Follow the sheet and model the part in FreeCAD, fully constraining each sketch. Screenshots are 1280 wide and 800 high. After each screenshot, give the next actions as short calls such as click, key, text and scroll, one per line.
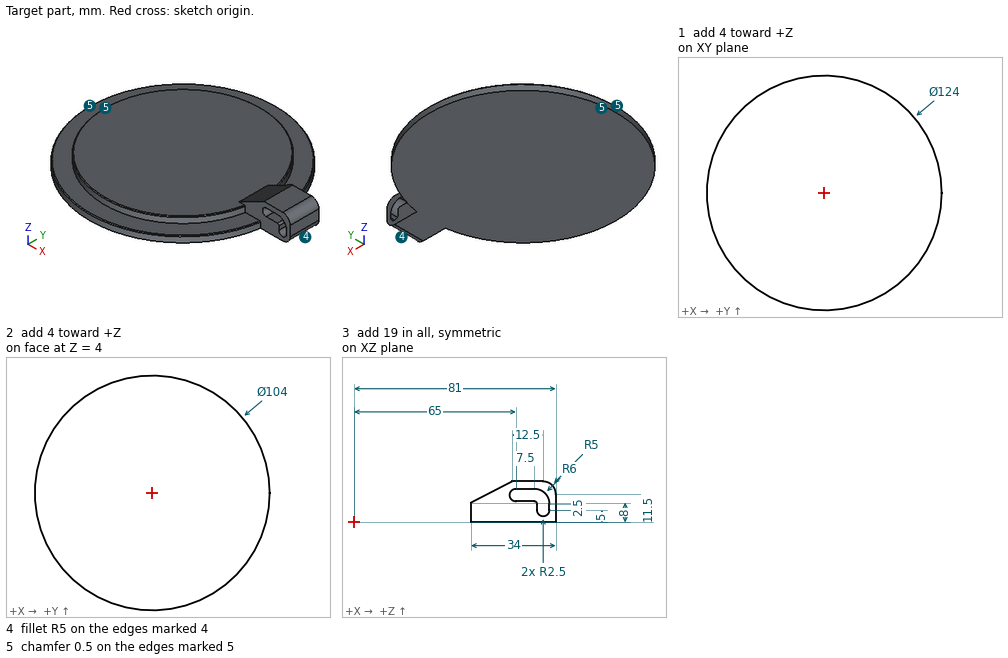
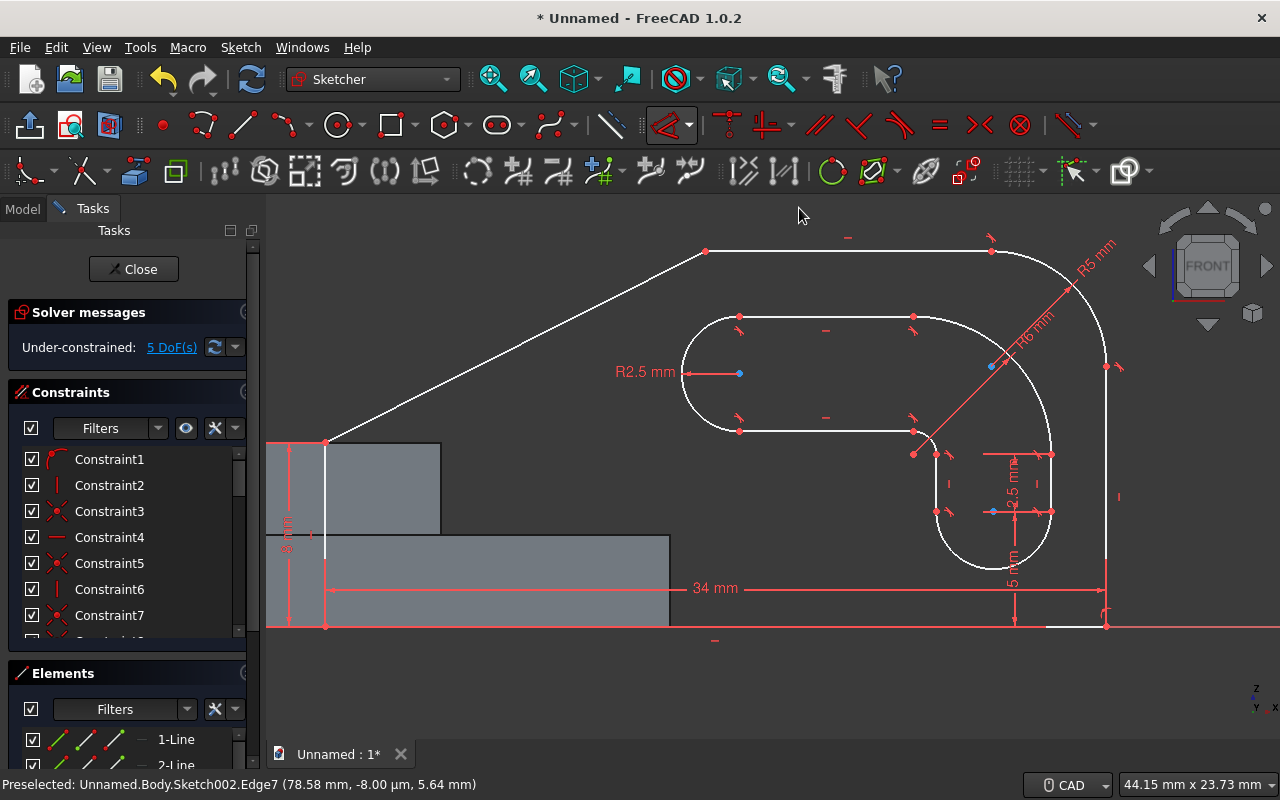
click(861, 317)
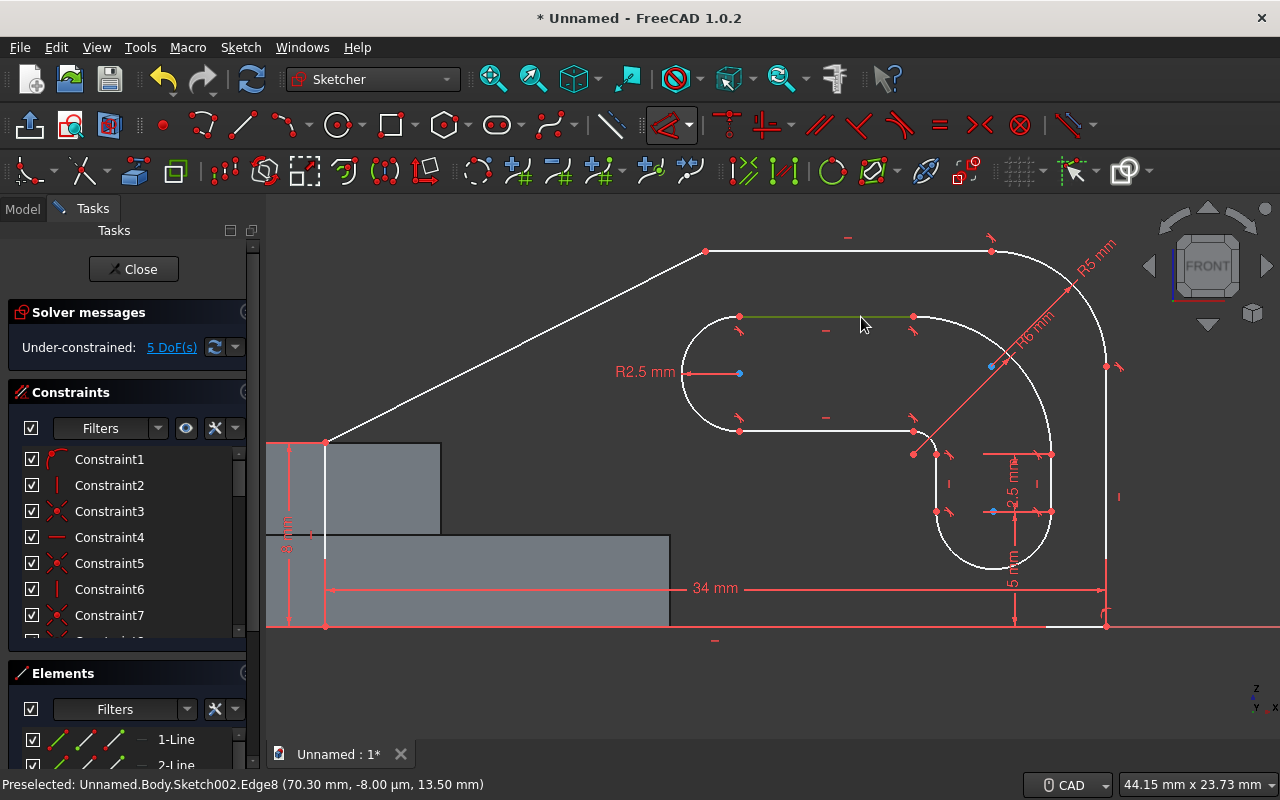
key(l)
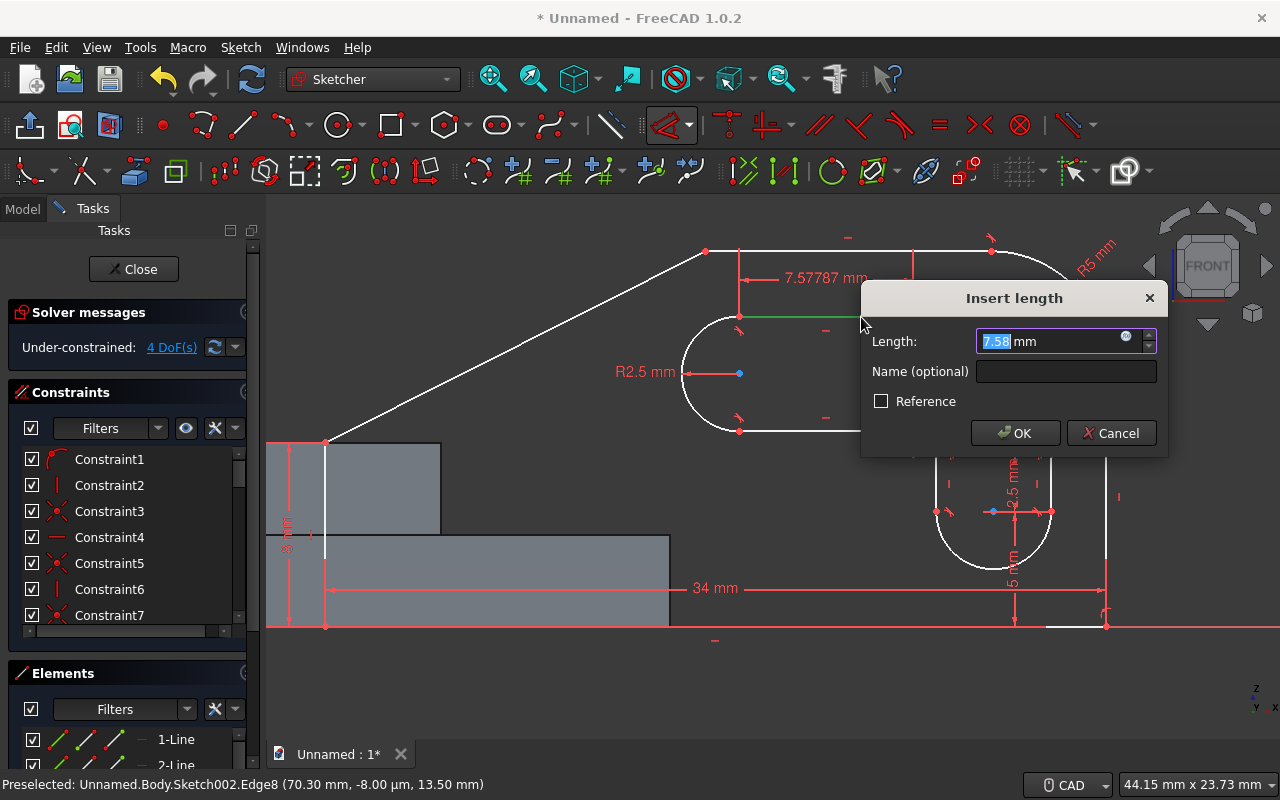
text(7.5)
key(Return)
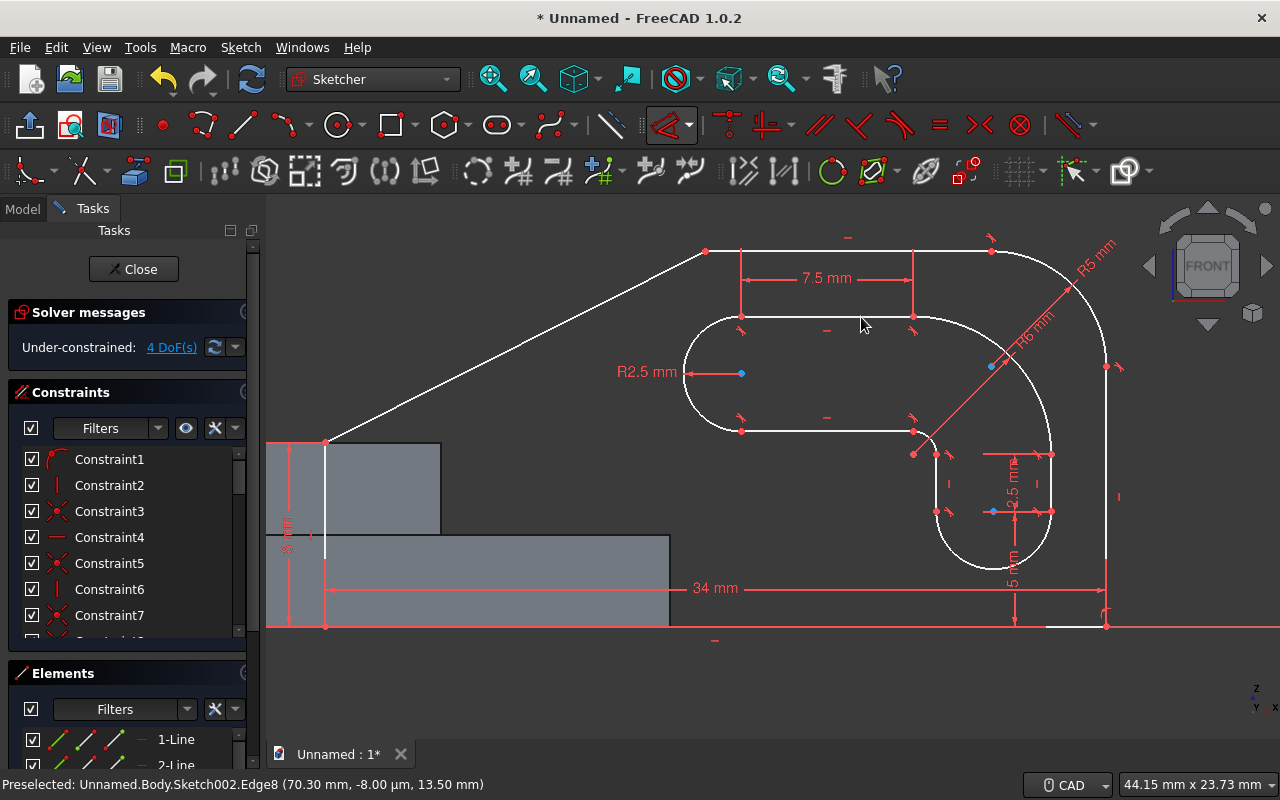
click(1106, 366)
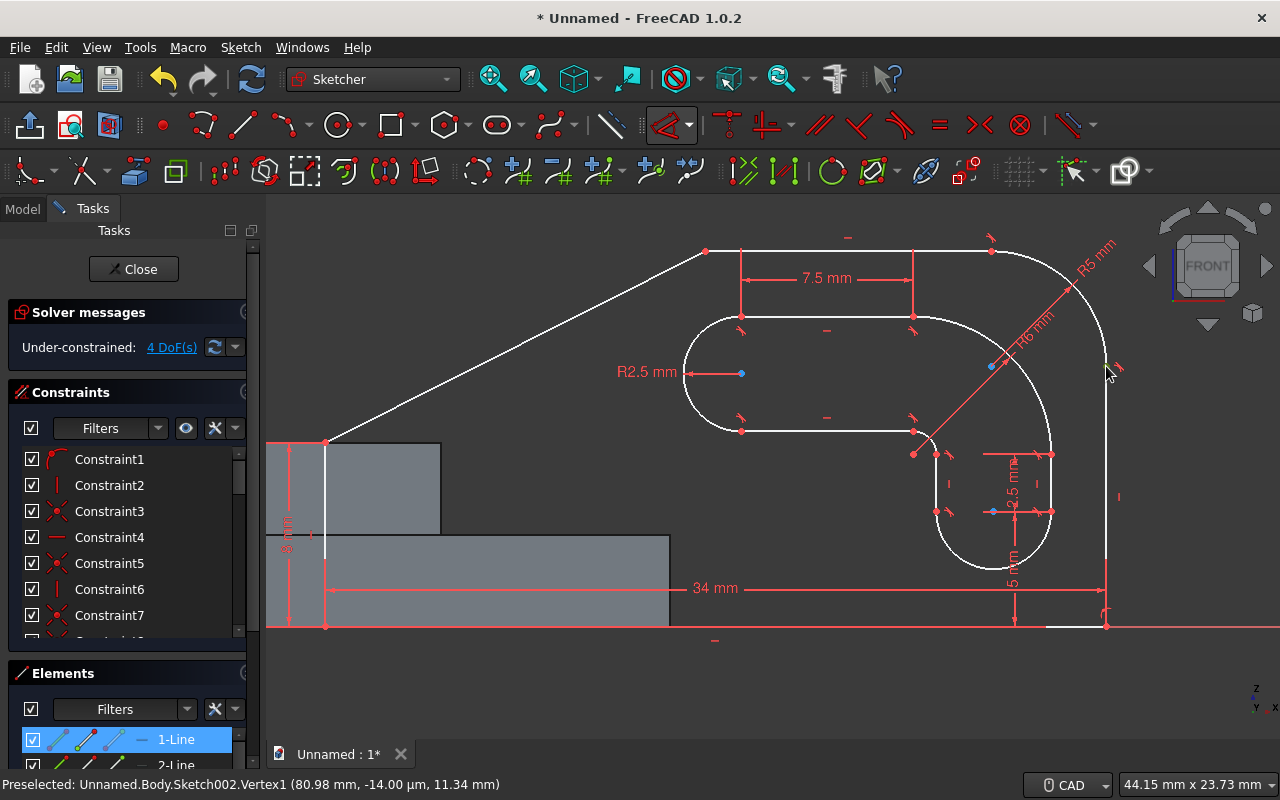
key(l)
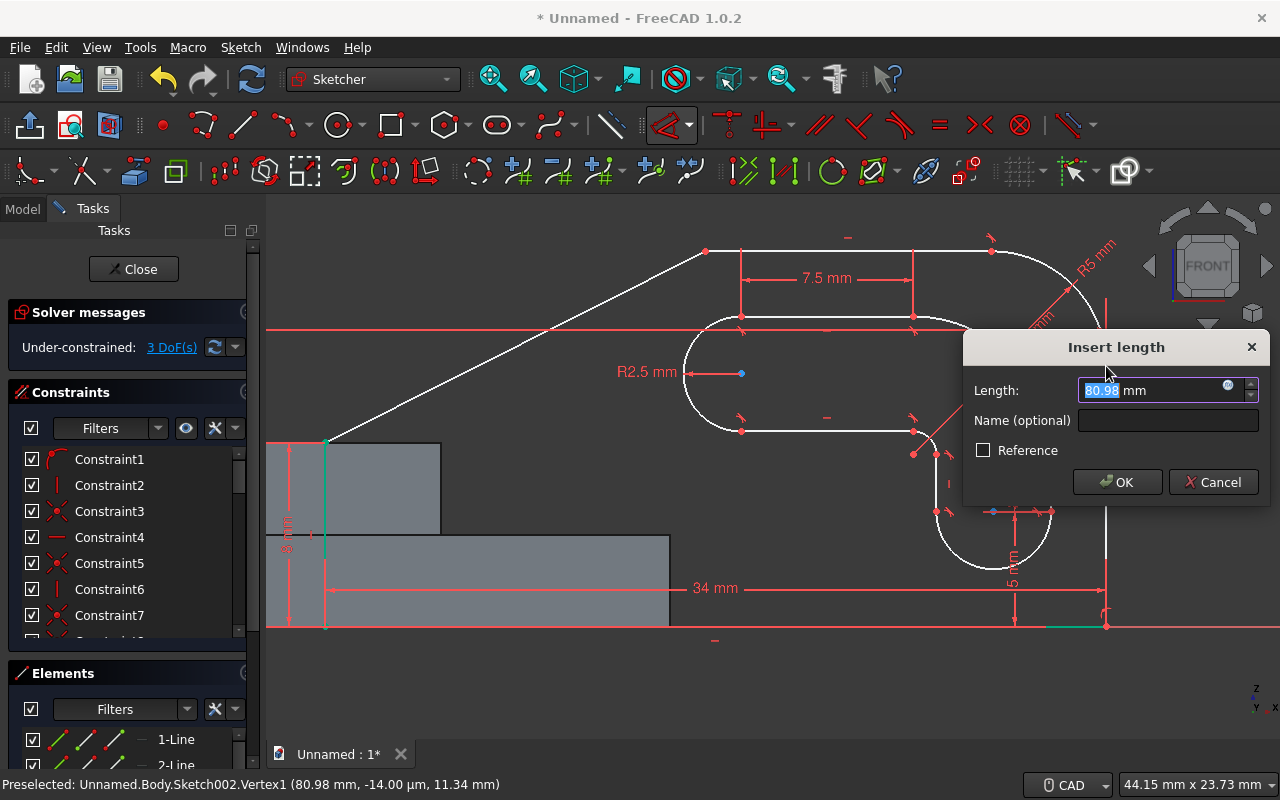
text(81)
key(Return)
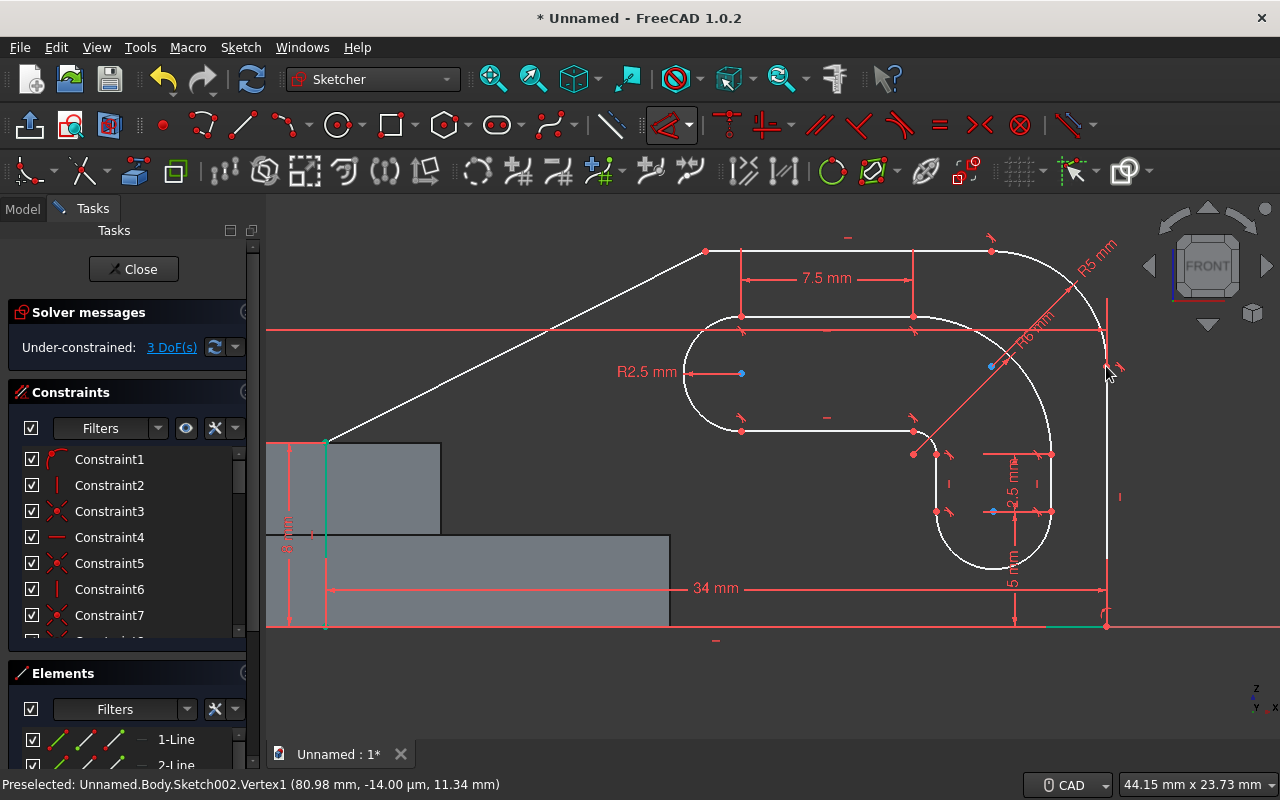
click(741, 317)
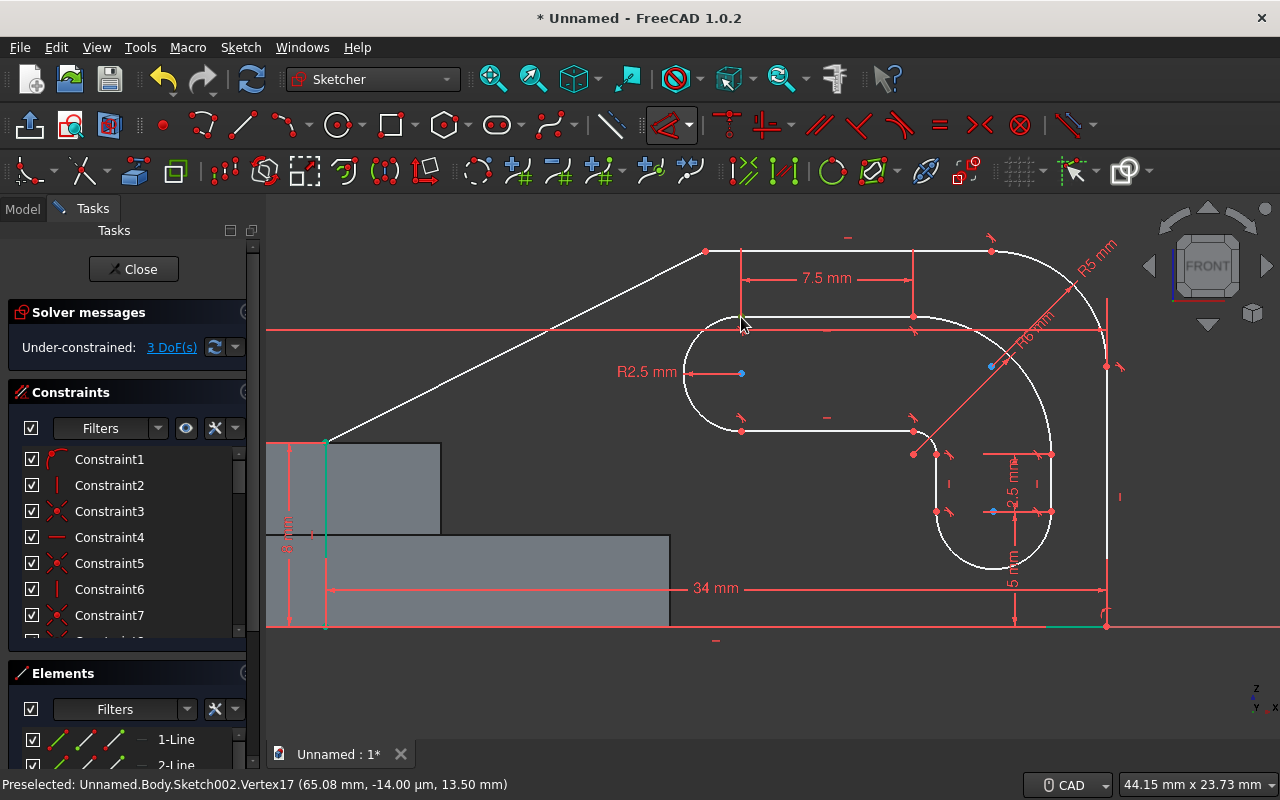
key(l)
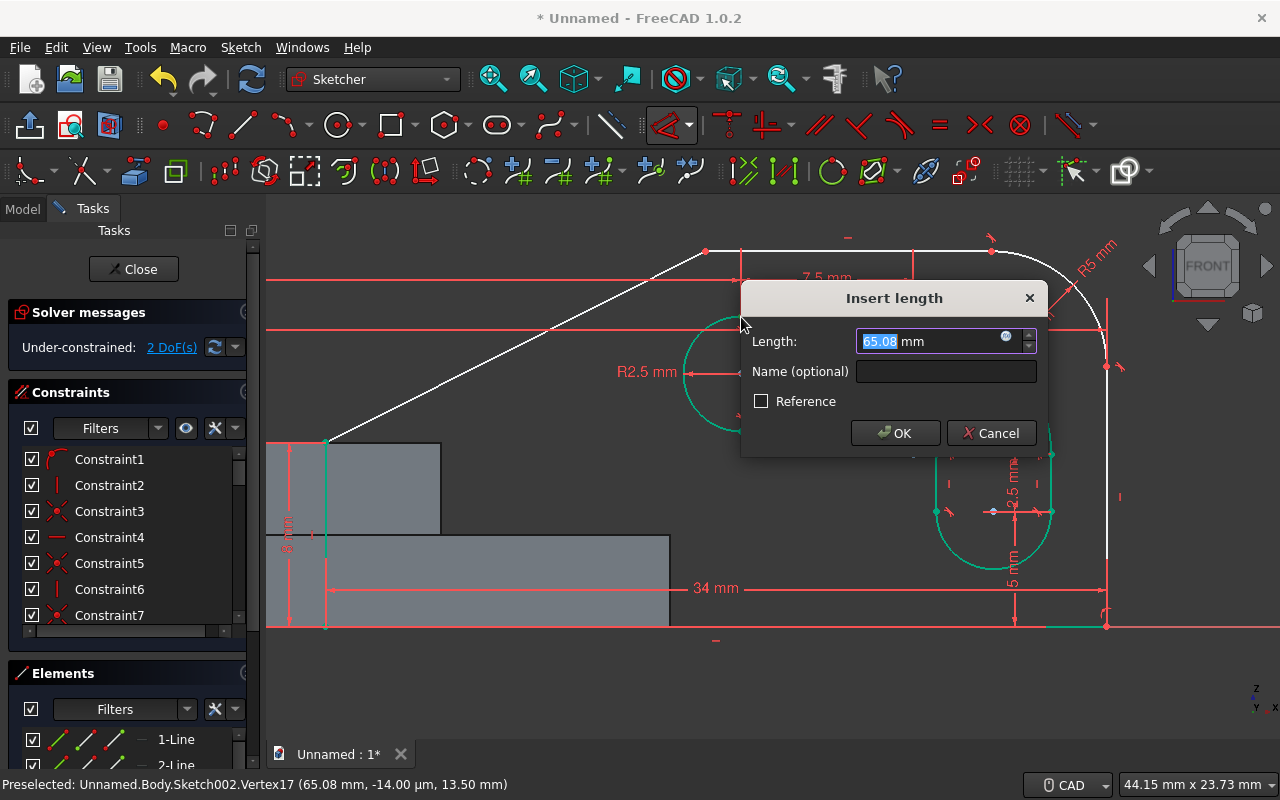
text(65)
key(Return)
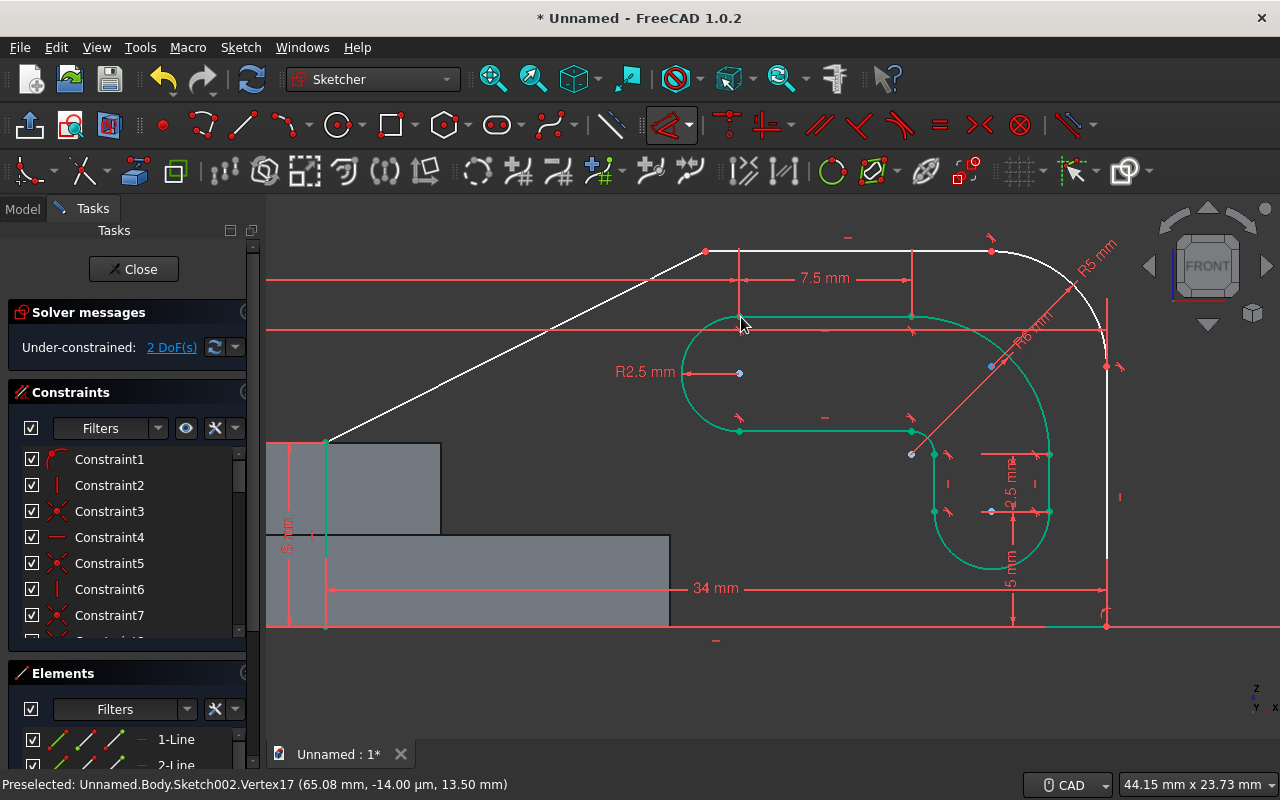
click(1107, 444)